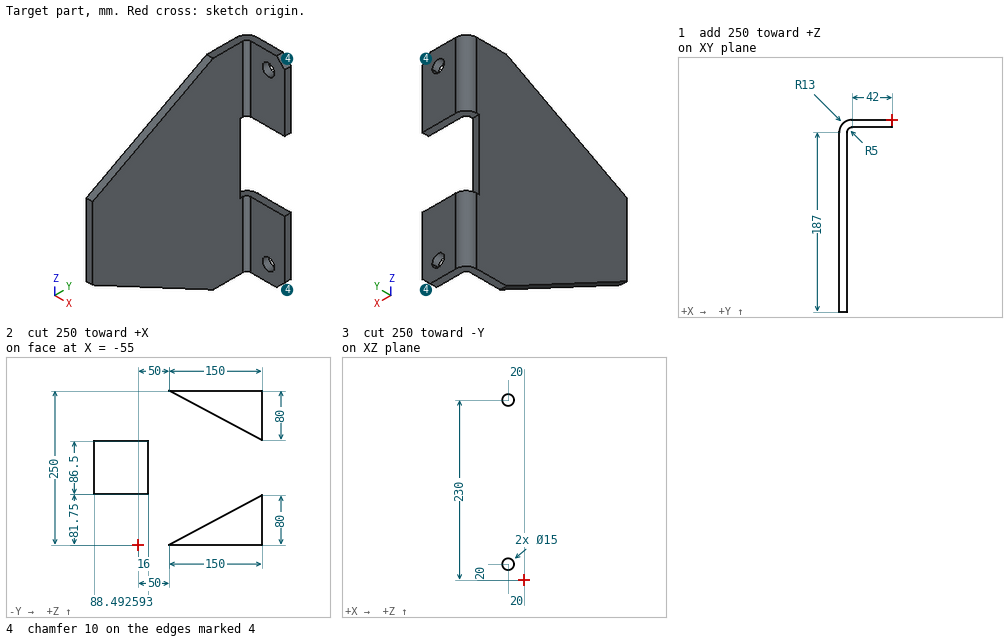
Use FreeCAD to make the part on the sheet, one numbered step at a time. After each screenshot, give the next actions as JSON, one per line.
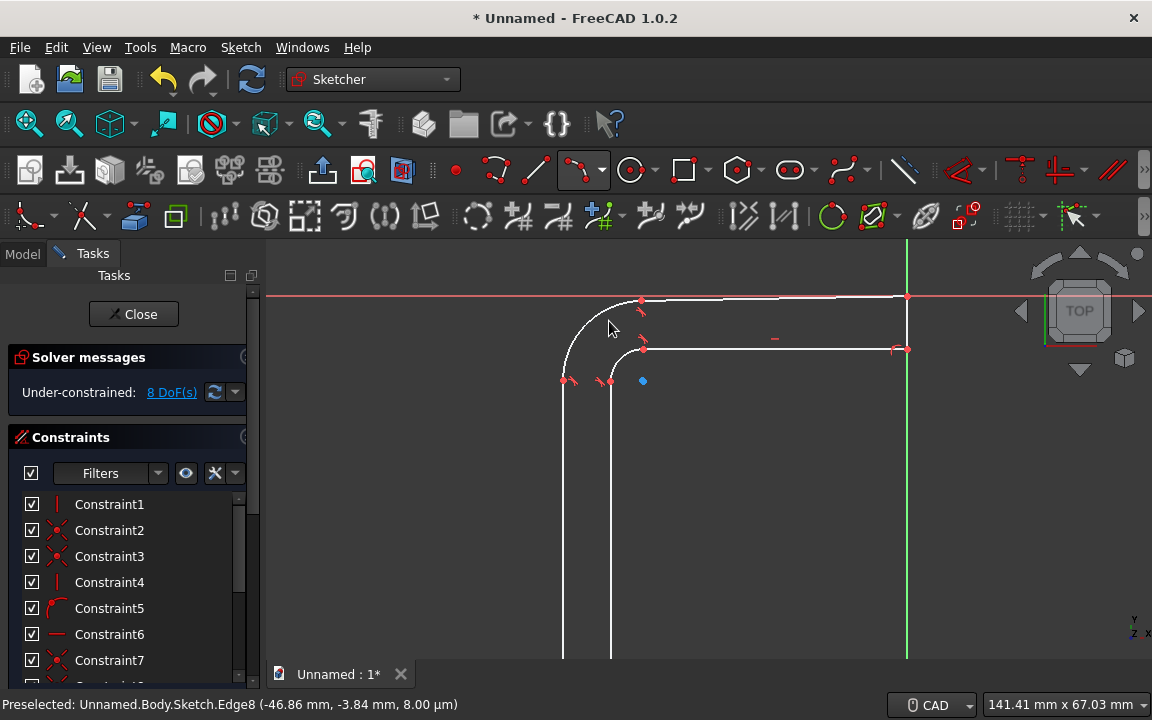
{"action": "scroll", "coordinate": [617, 329], "scroll_direction": "down", "scroll_amount": 8}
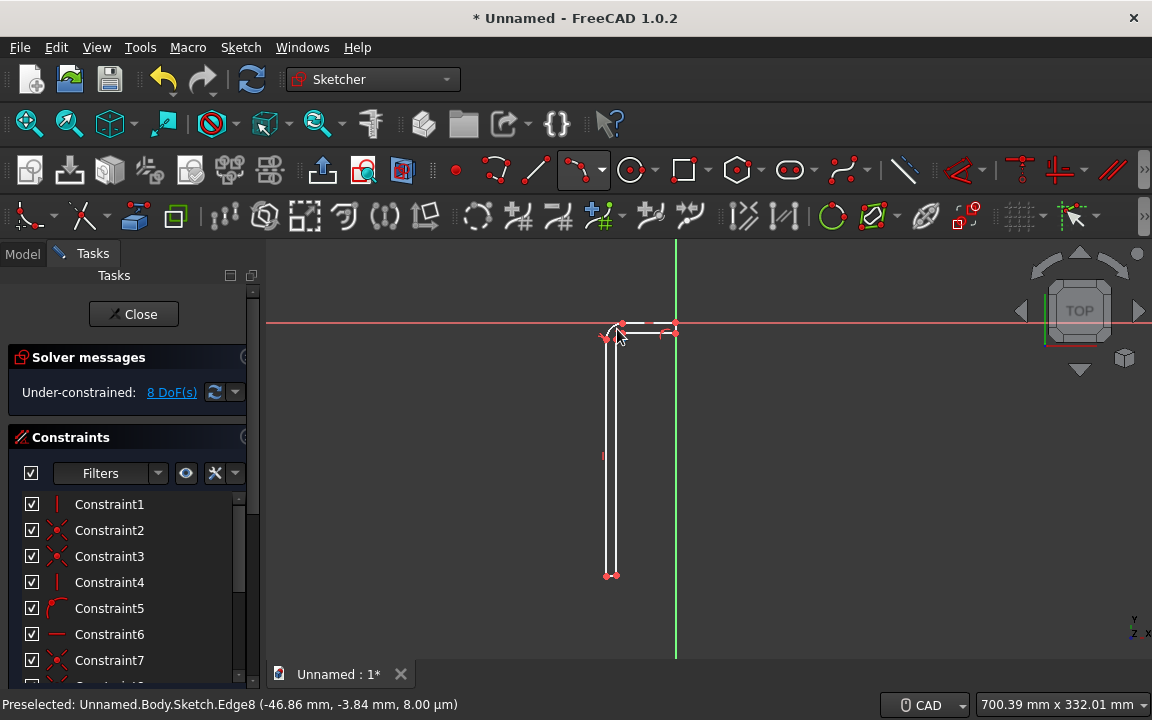
{"action": "scroll", "coordinate": [609, 576], "scroll_direction": "up", "scroll_amount": 8}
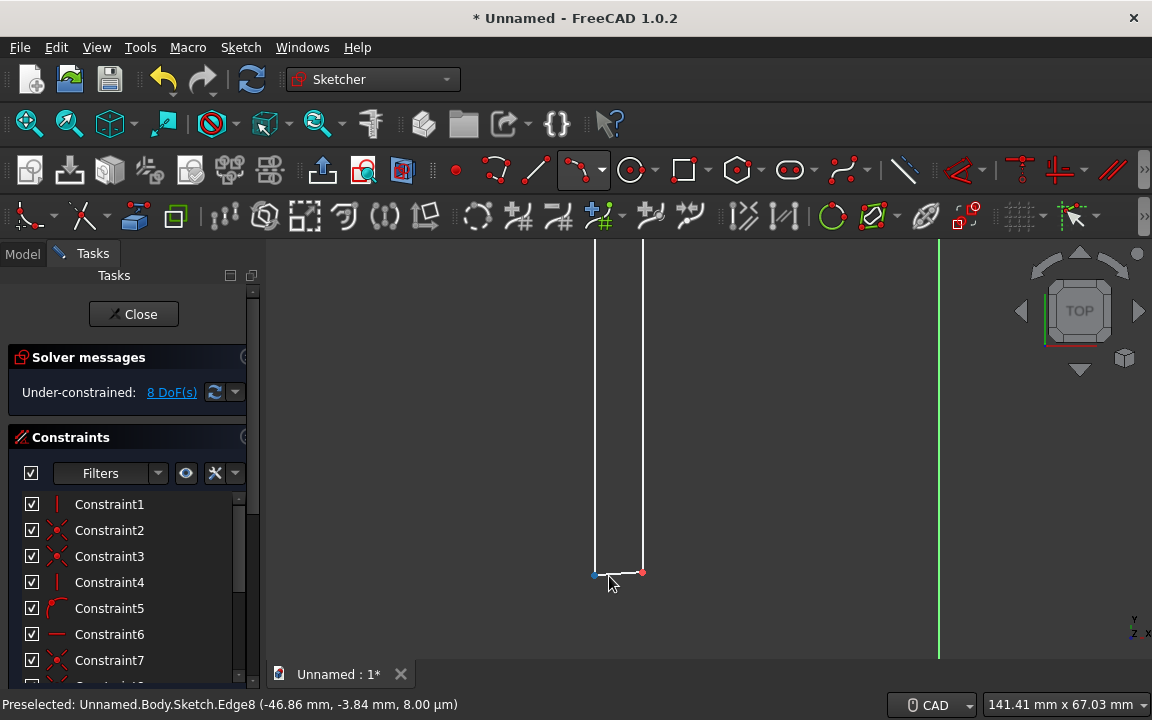
{"action": "left_click", "coordinate": [609, 574]}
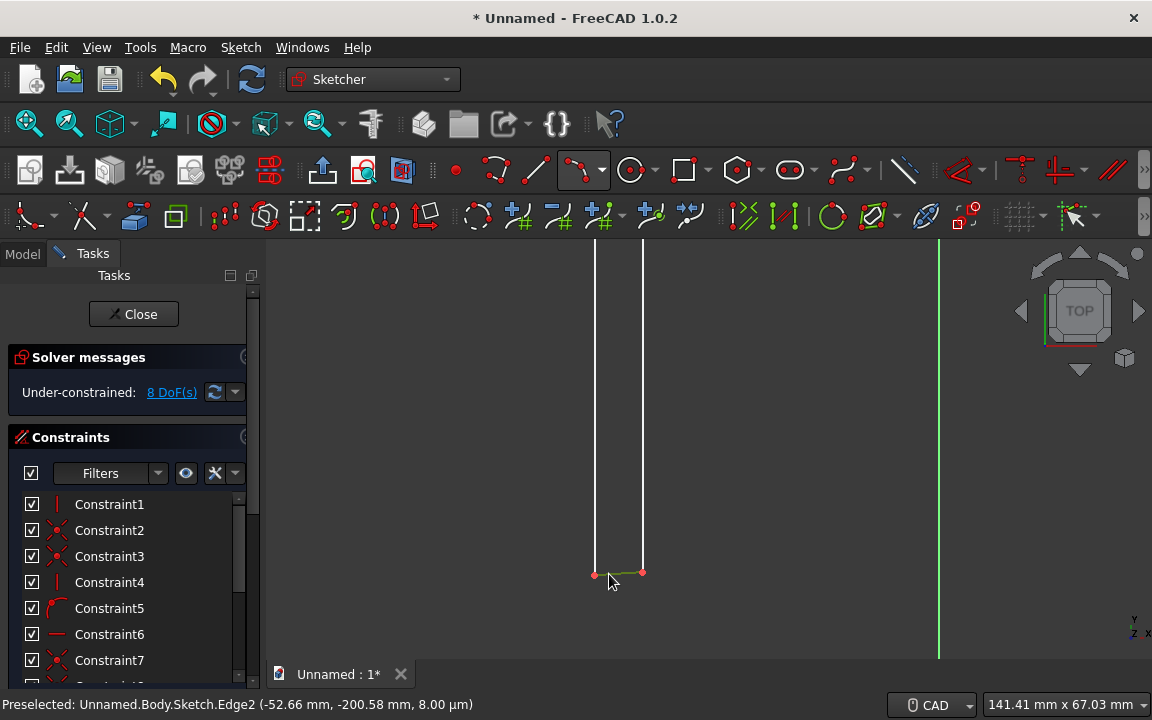
{"action": "key", "text": "h"}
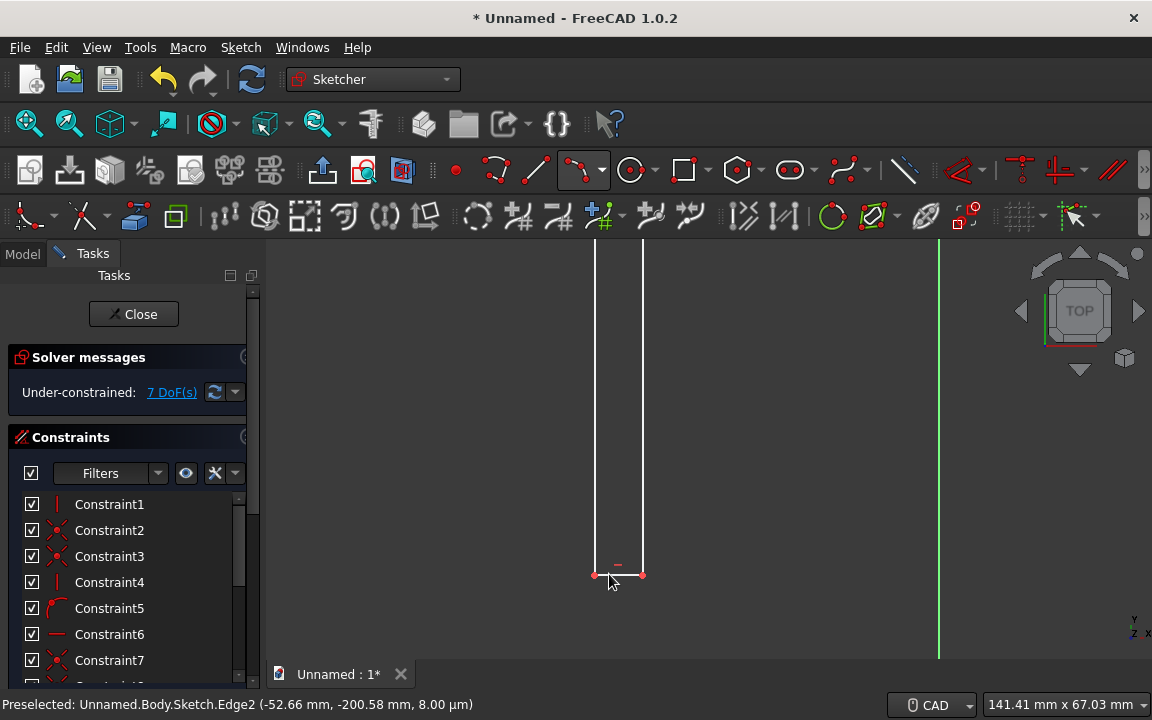
{"action": "scroll", "coordinate": [609, 577], "scroll_direction": "down", "scroll_amount": 8}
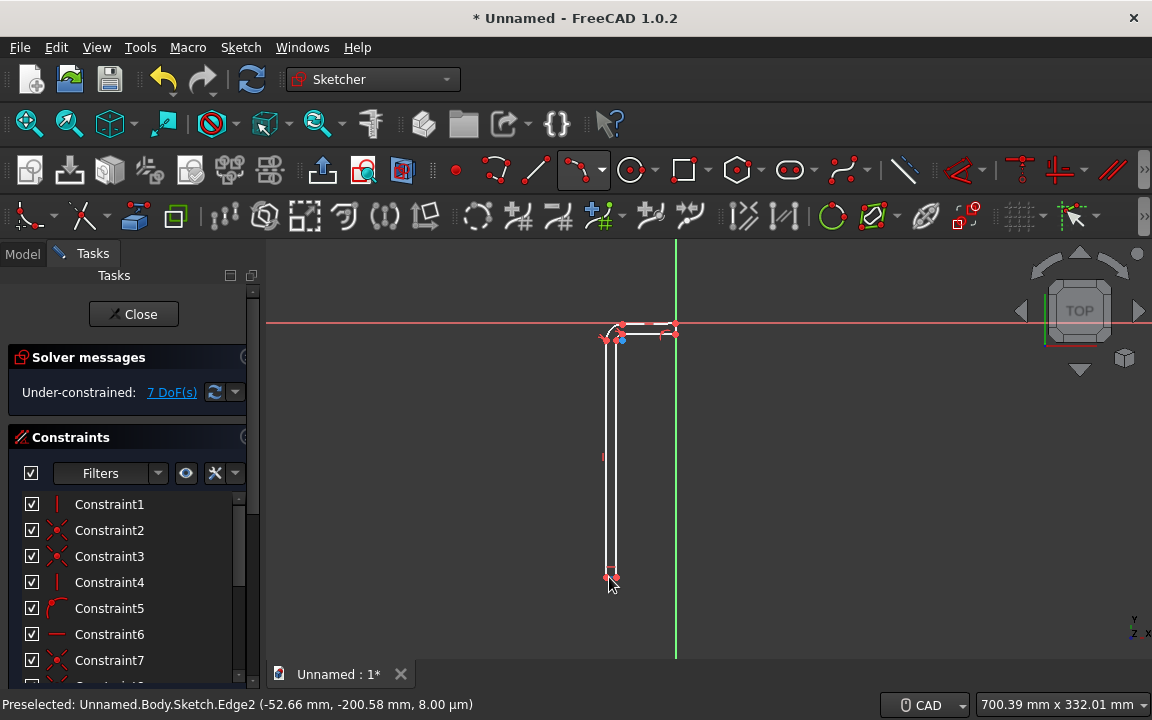
{"action": "scroll", "coordinate": [660, 324], "scroll_direction": "up", "scroll_amount": 2}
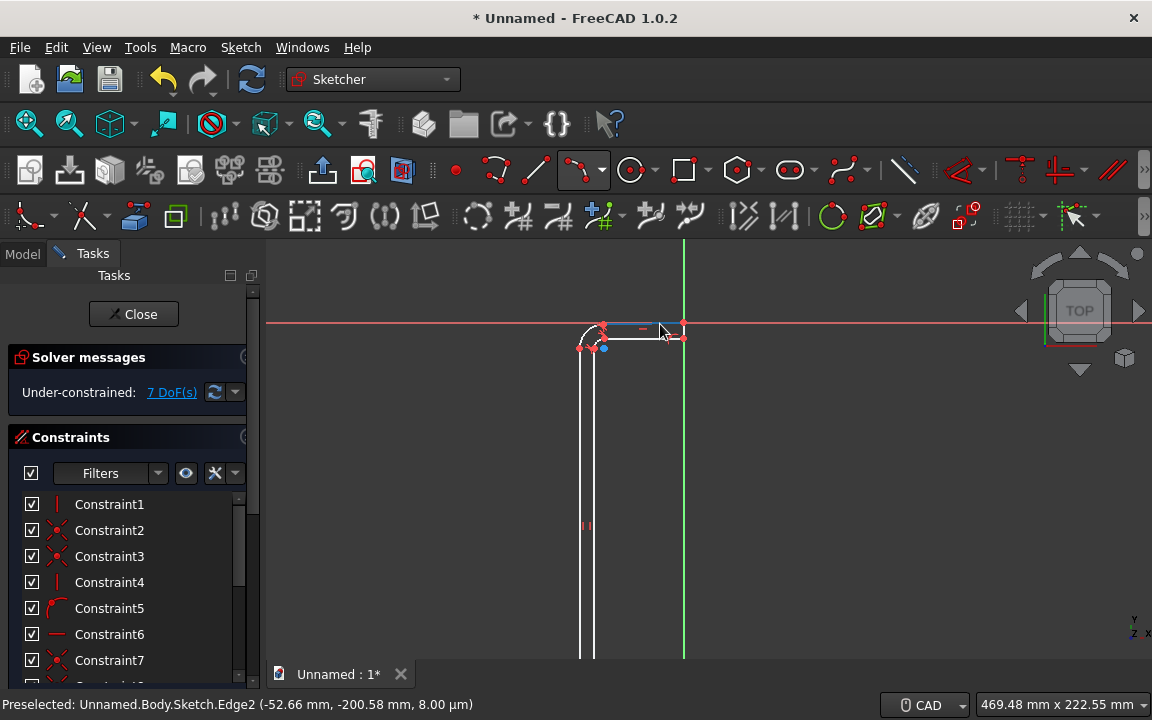
{"action": "left_click", "coordinate": [660, 323]}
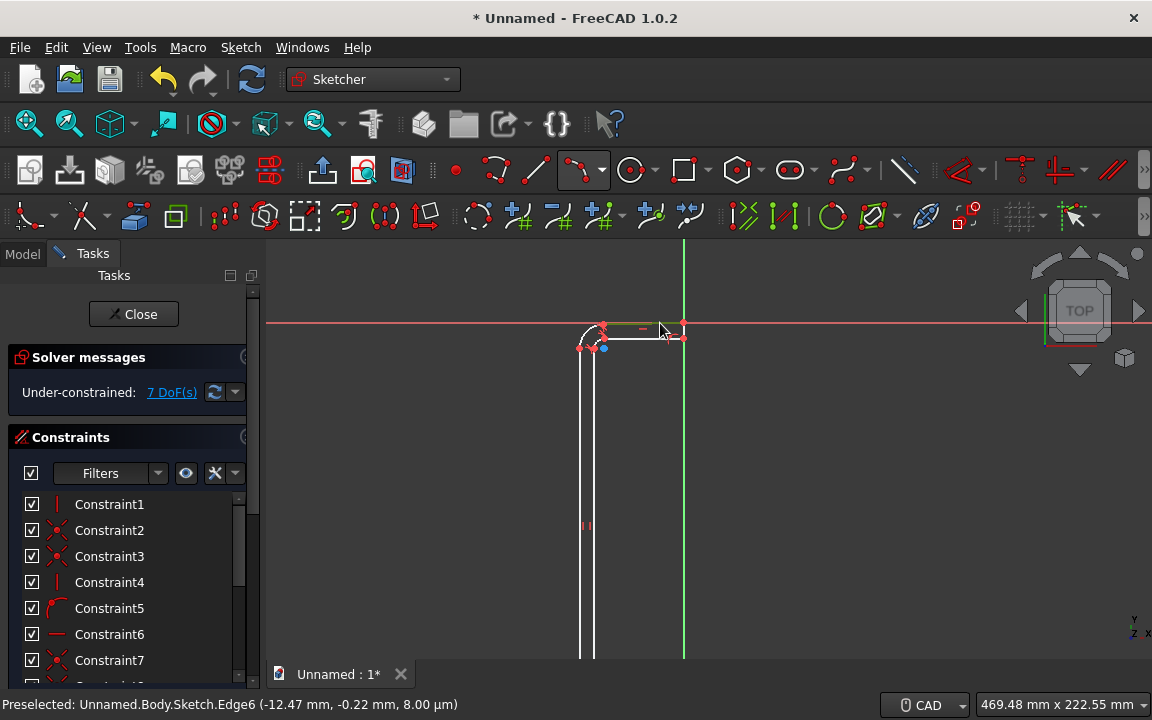
{"action": "key", "text": "h"}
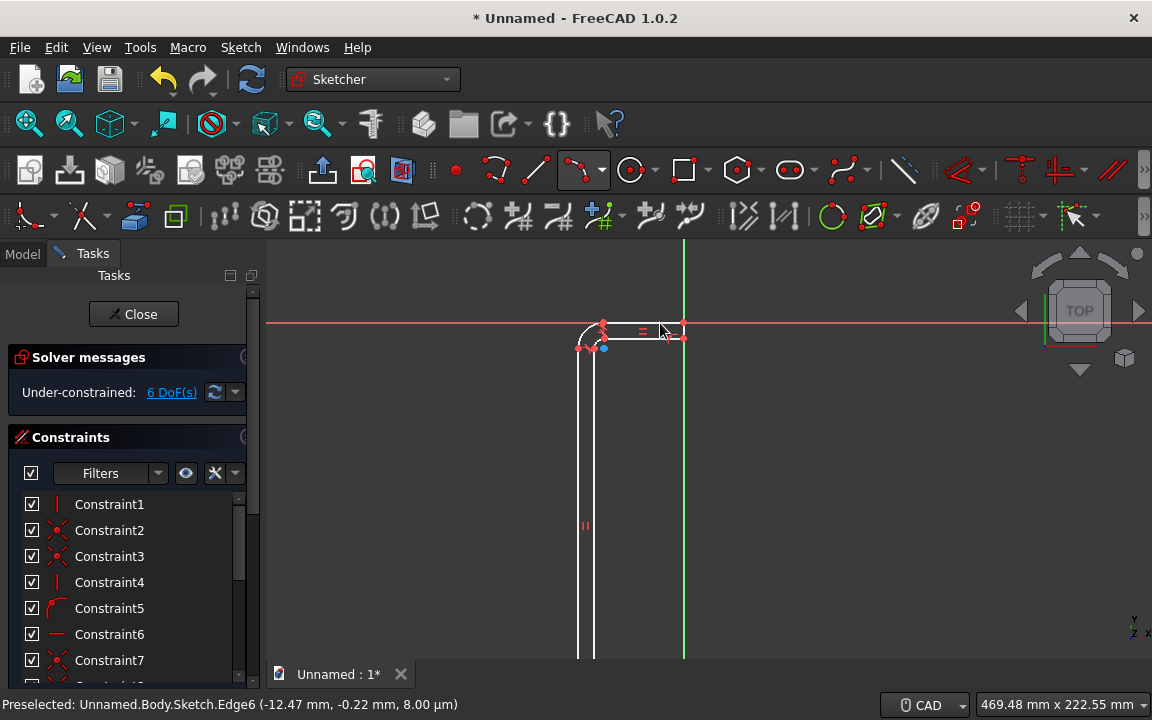
{"action": "scroll", "coordinate": [597, 342], "scroll_direction": "up", "scroll_amount": 4}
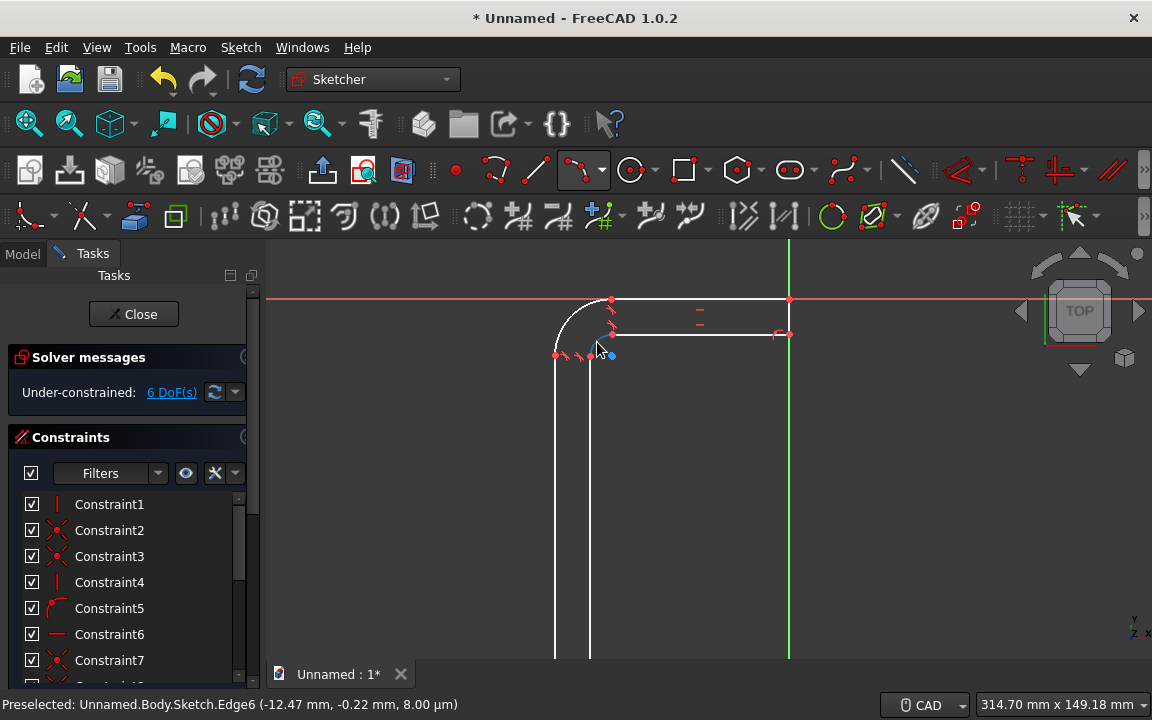
{"action": "left_click", "coordinate": [597, 341]}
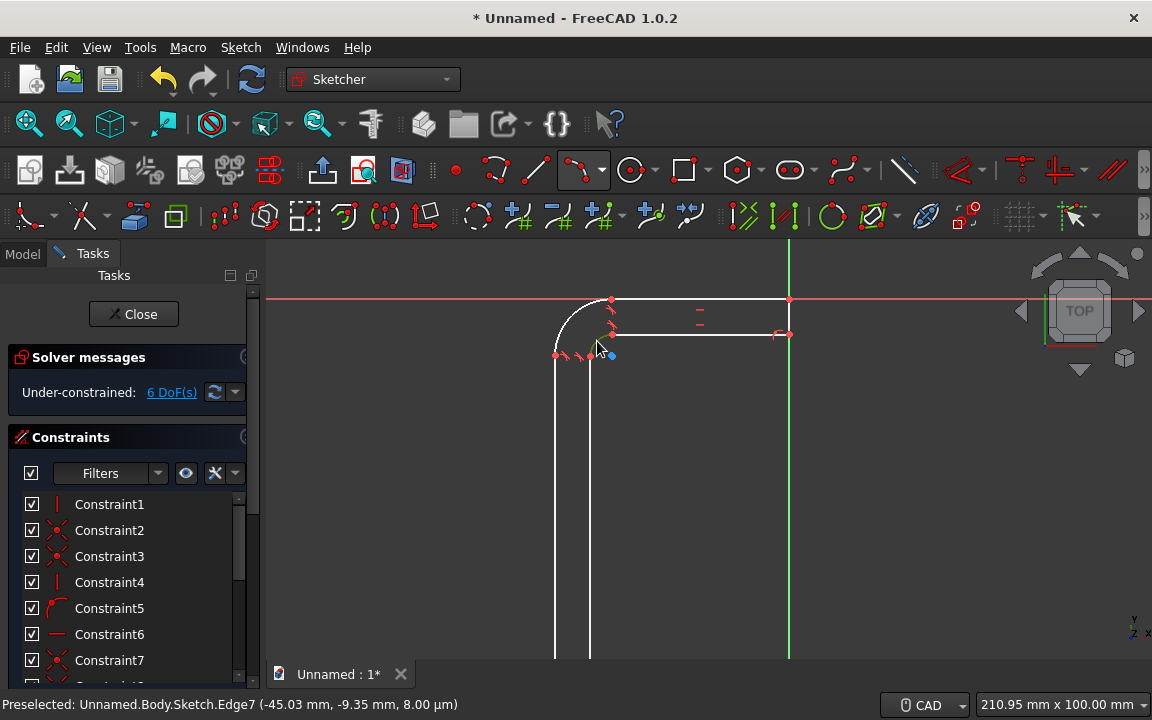
{"action": "left_click", "coordinate": [561, 330]}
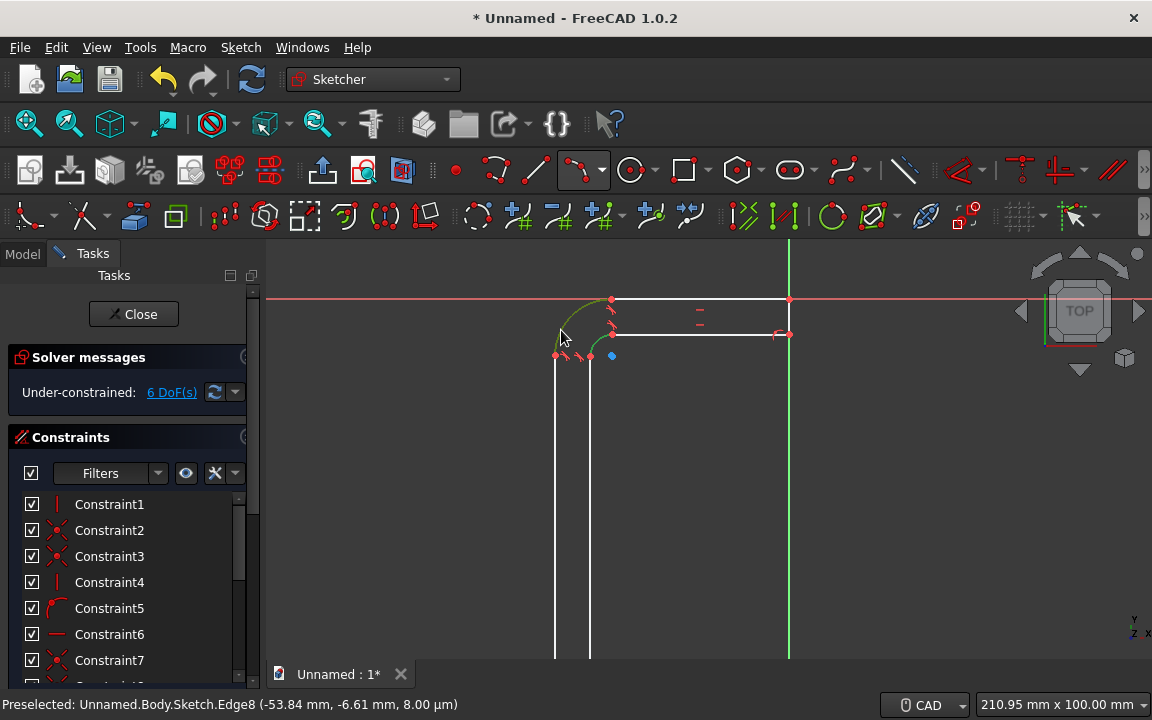
{"action": "key", "text": "c"}